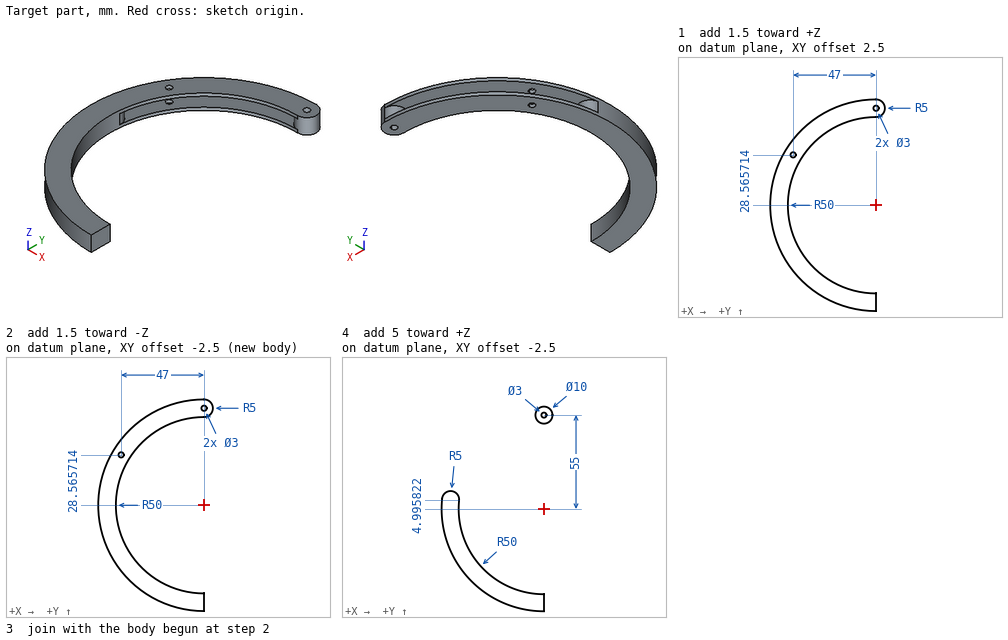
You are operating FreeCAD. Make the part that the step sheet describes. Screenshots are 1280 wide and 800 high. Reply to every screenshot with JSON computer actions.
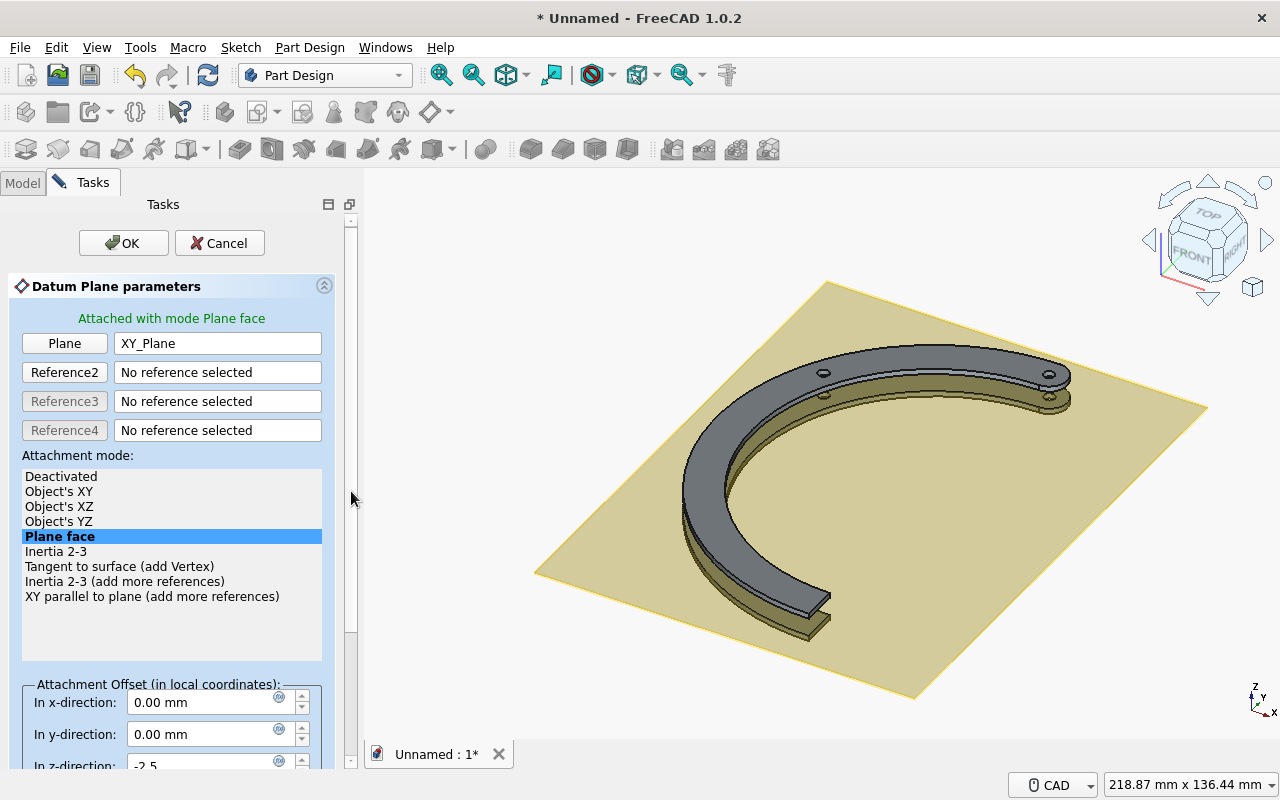
{"action": "left_click", "coordinate": [124, 243]}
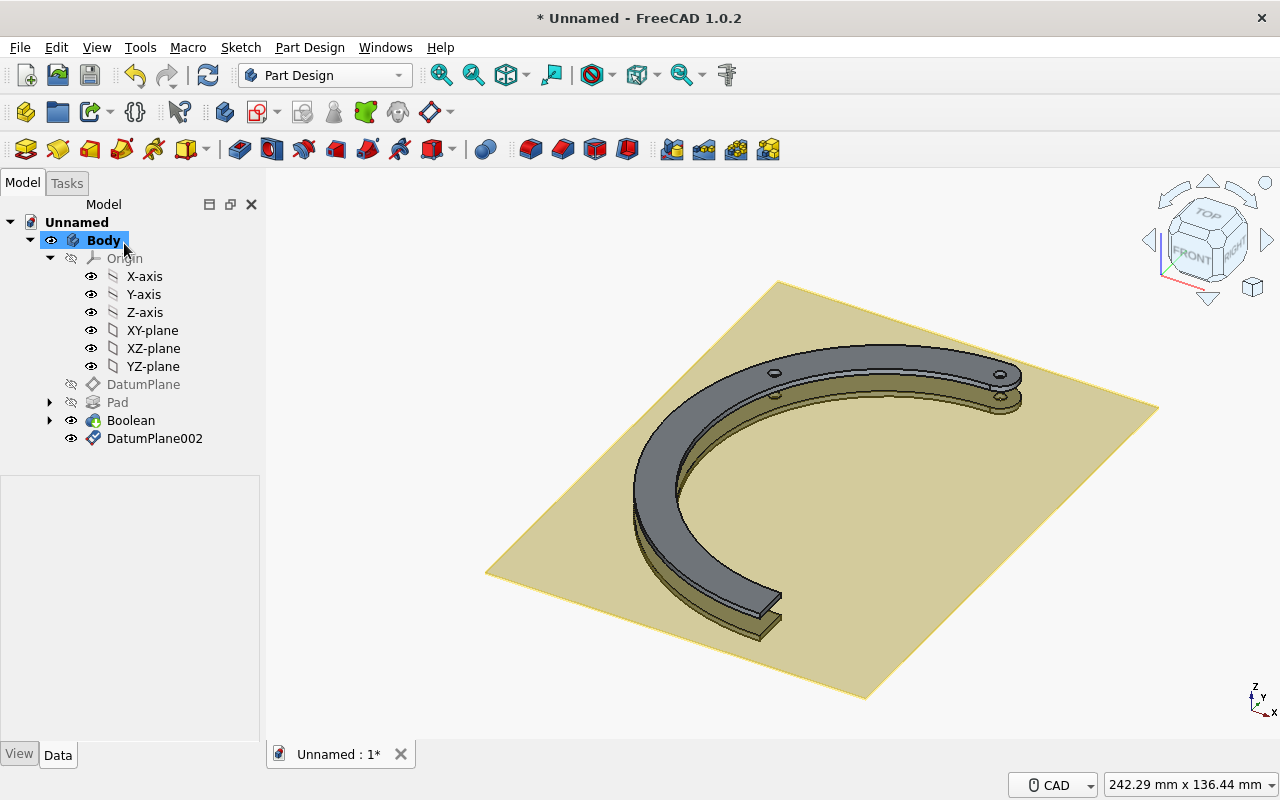
{"action": "left_click", "coordinate": [116, 438]}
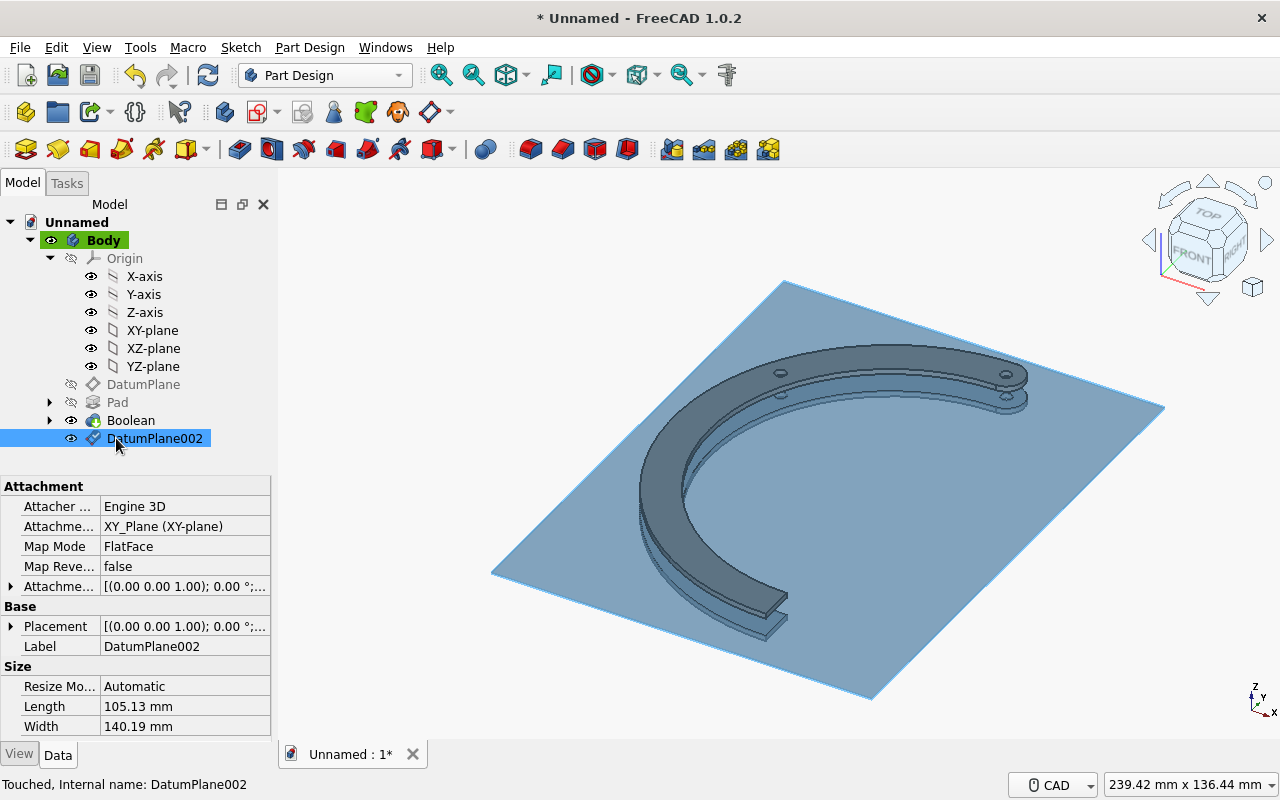
{"action": "left_click", "coordinate": [258, 112]}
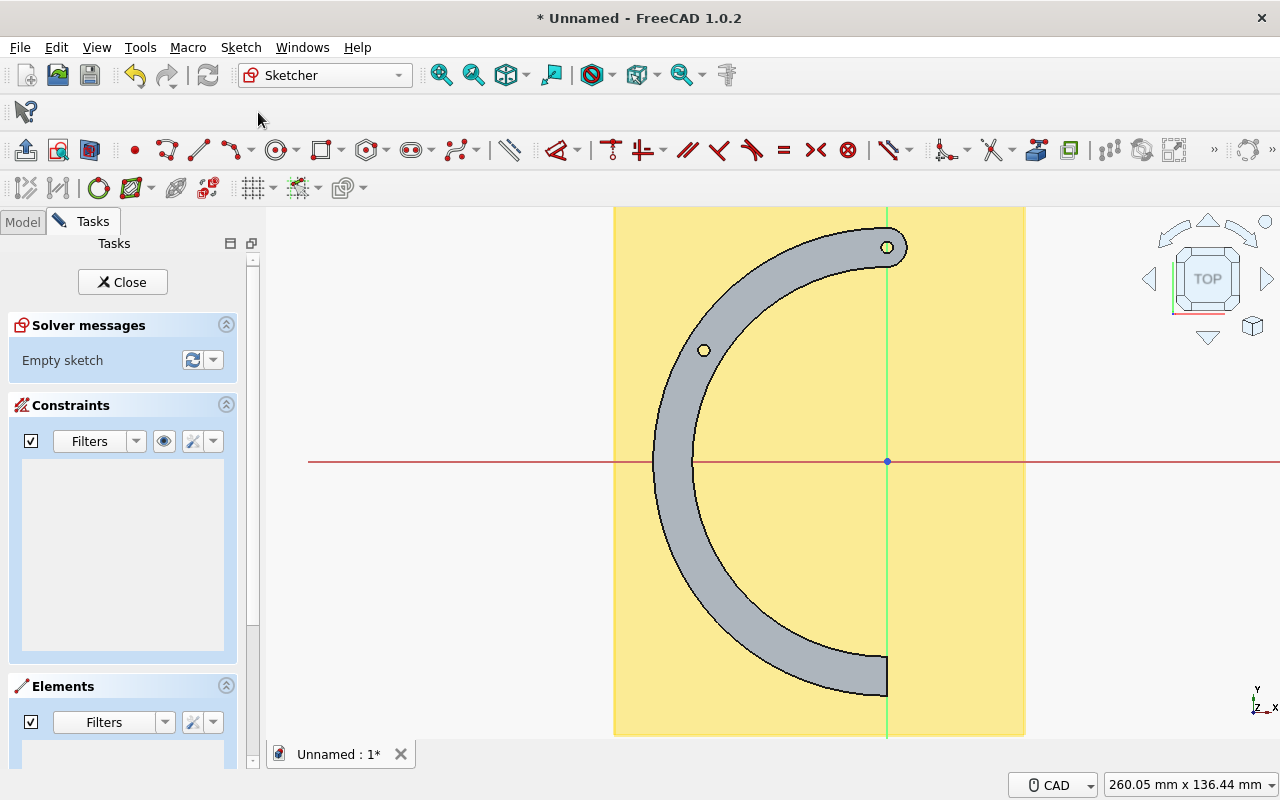
{"action": "left_click", "coordinate": [90, 150]}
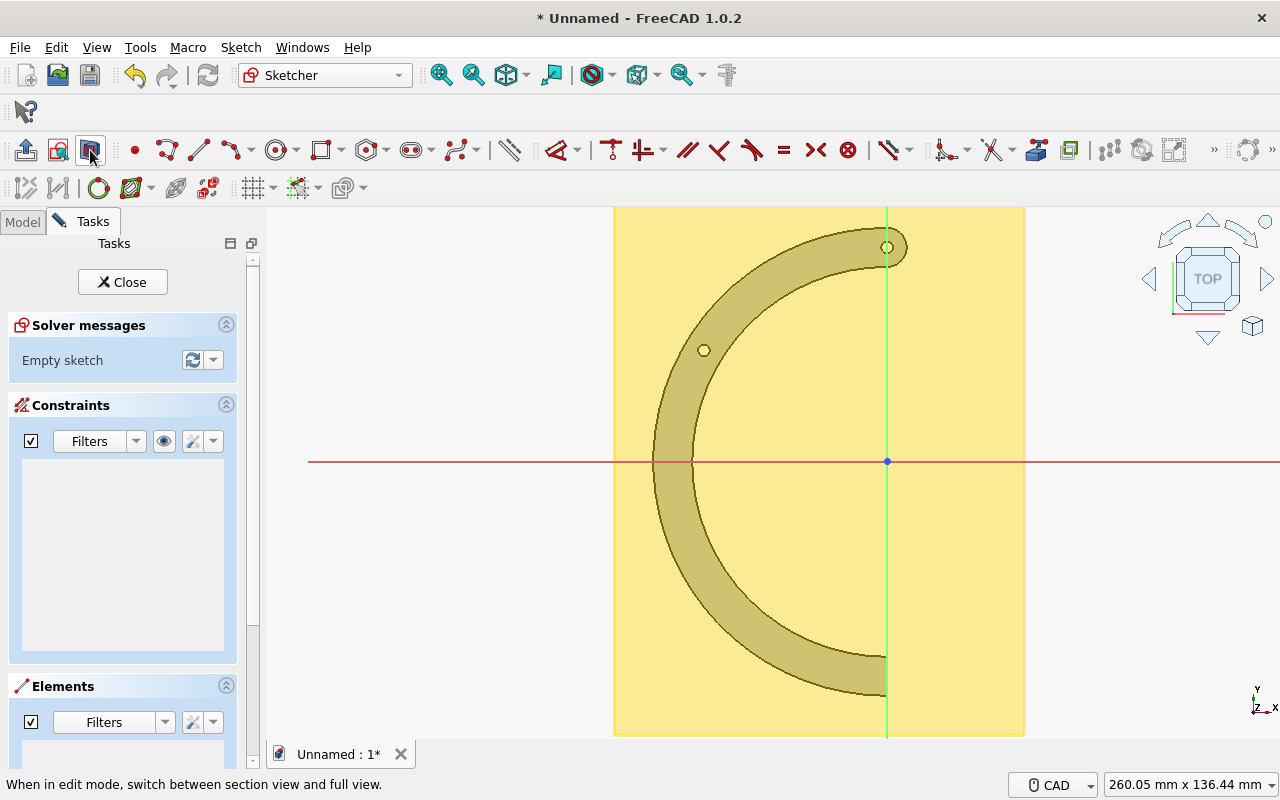
{"action": "scroll", "coordinate": [550, 496], "scroll_direction": "down", "scroll_amount": 2}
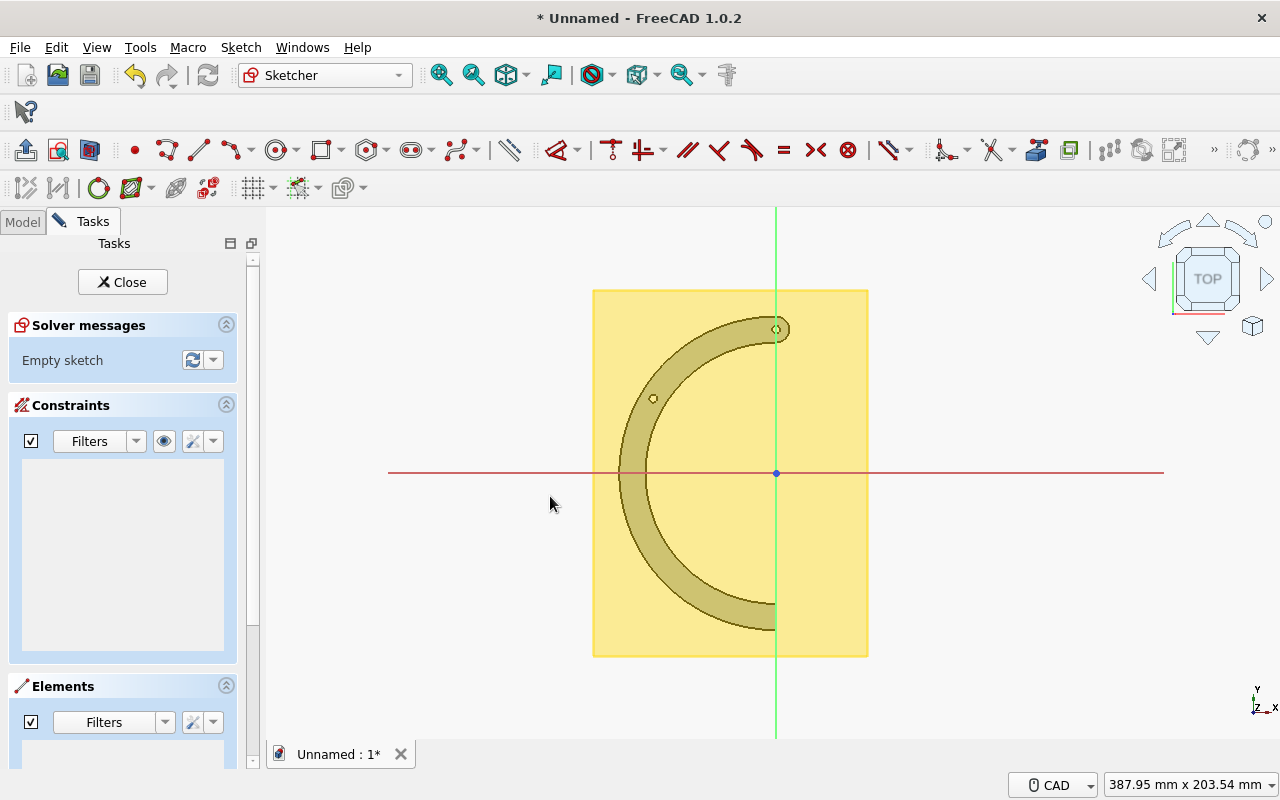
{"action": "left_click", "coordinate": [200, 150]}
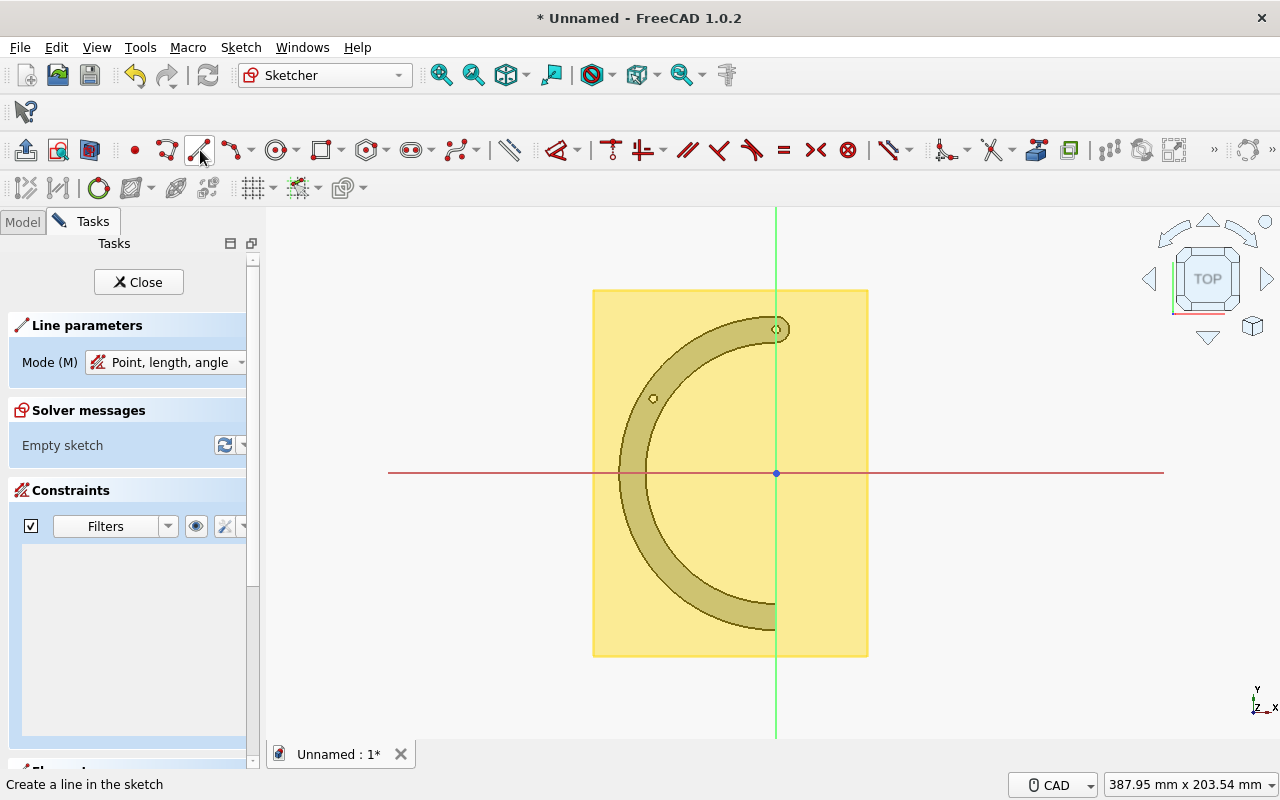
{"action": "left_click", "coordinate": [776, 630]}
{"action": "left_click", "coordinate": [767, 604]}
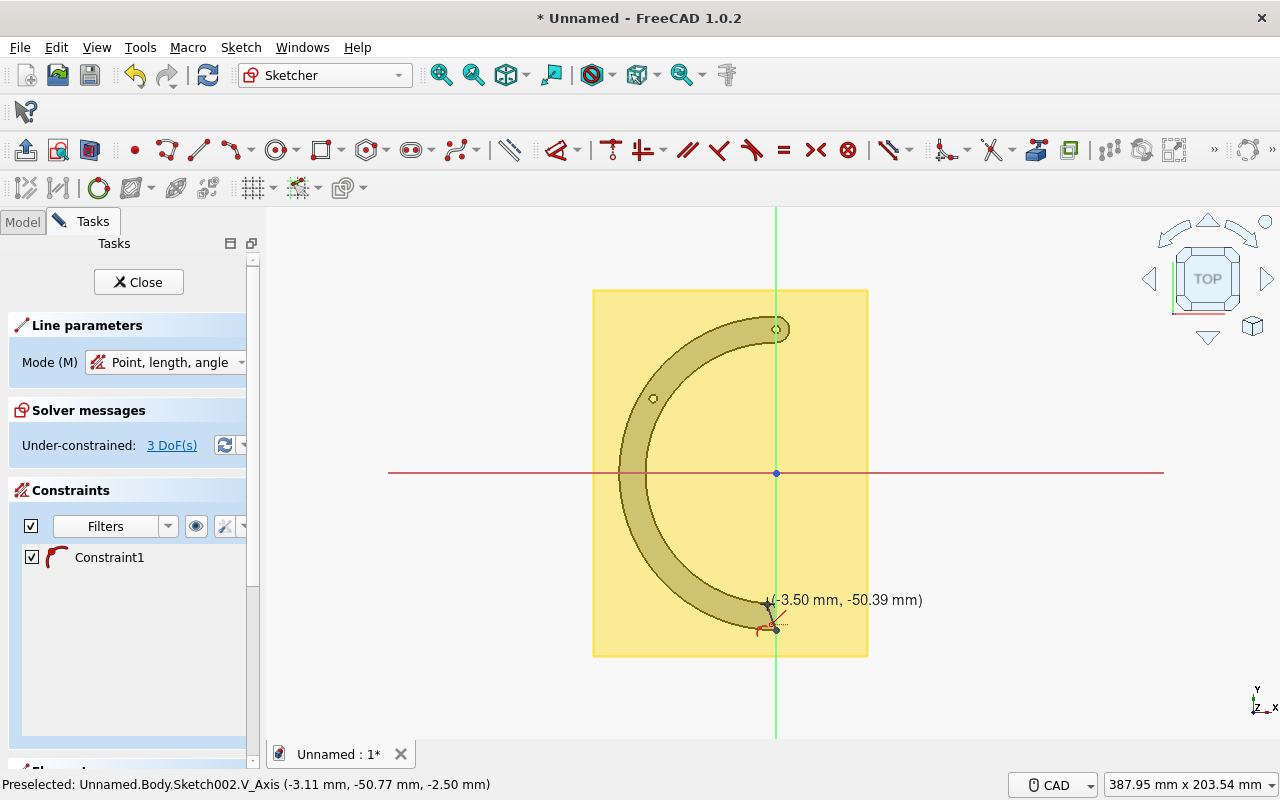
{"action": "left_click", "coordinate": [232, 150]}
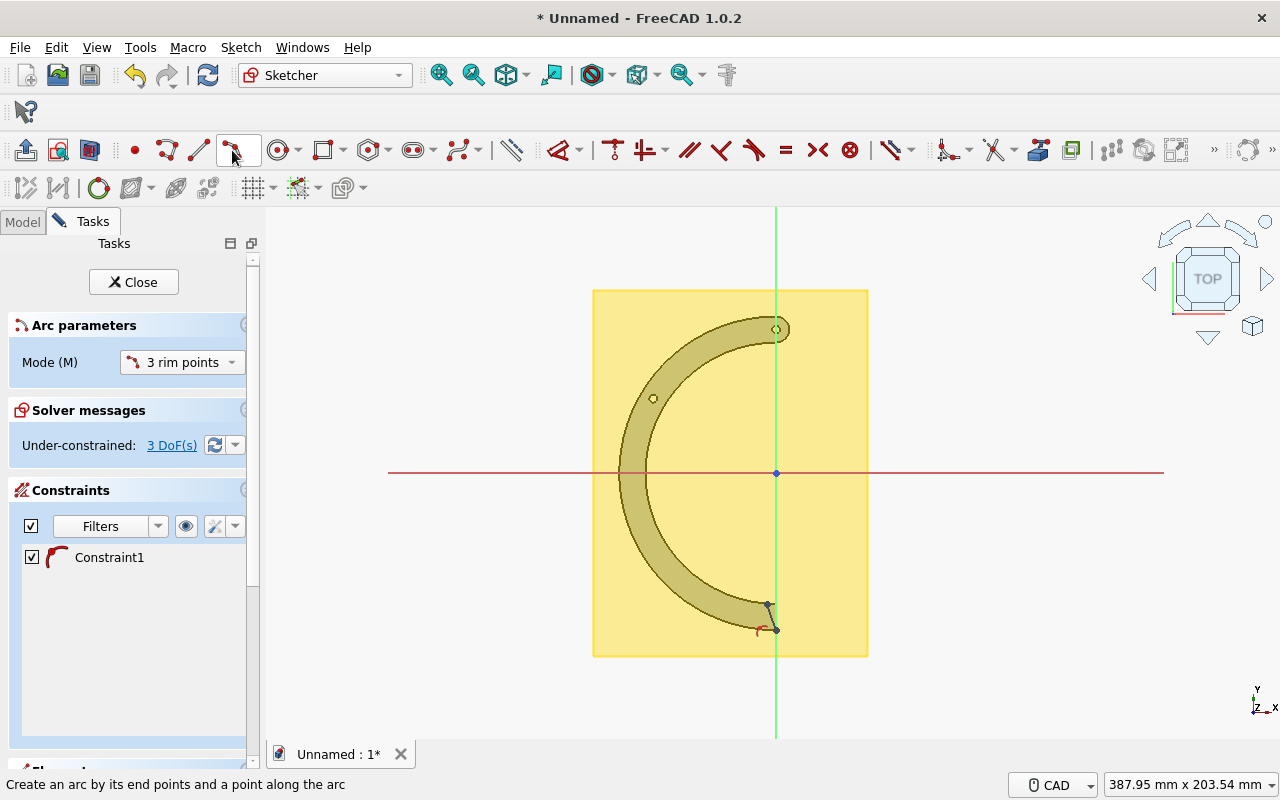
{"action": "left_click", "coordinate": [767, 605]}
{"action": "left_click", "coordinate": [646, 460]}
{"action": "left_click", "coordinate": [679, 561]}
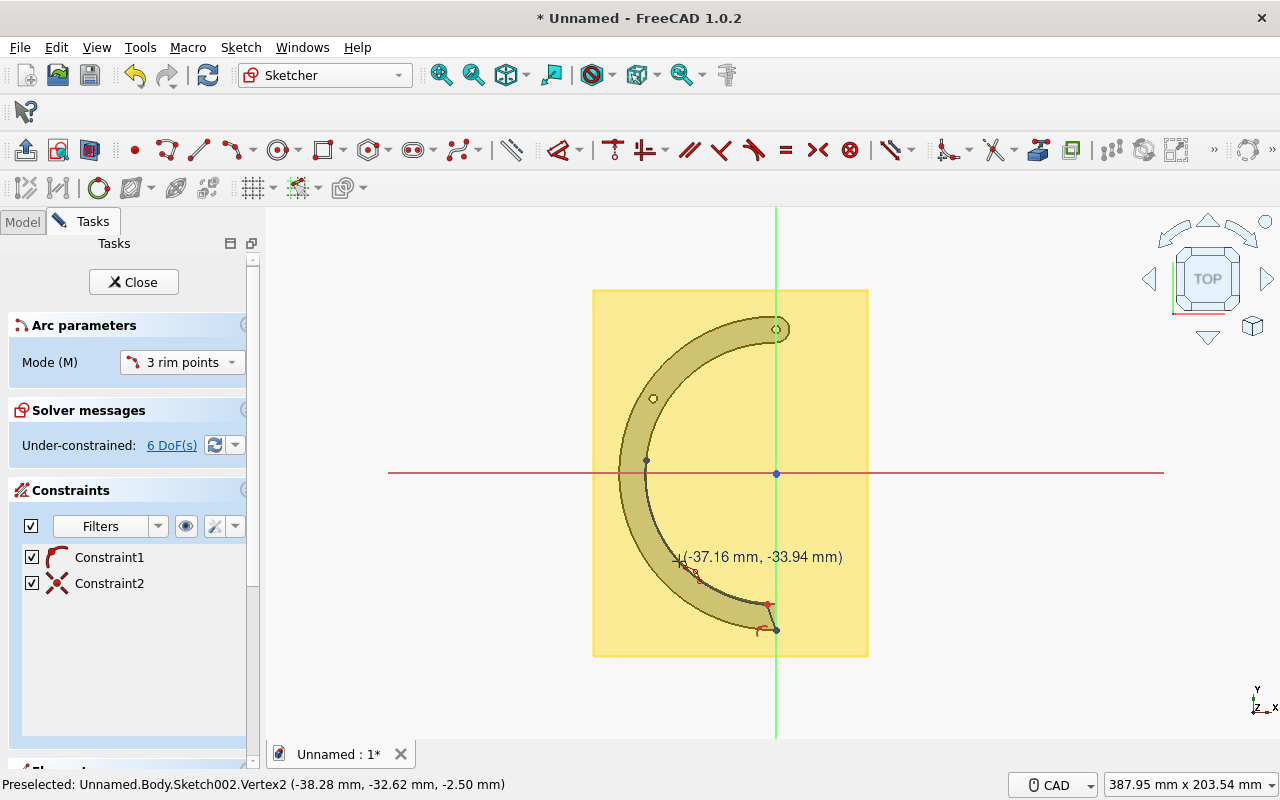
{"action": "left_click", "coordinate": [646, 461]}
{"action": "left_click", "coordinate": [620, 458]}
{"action": "left_click", "coordinate": [634, 446]}